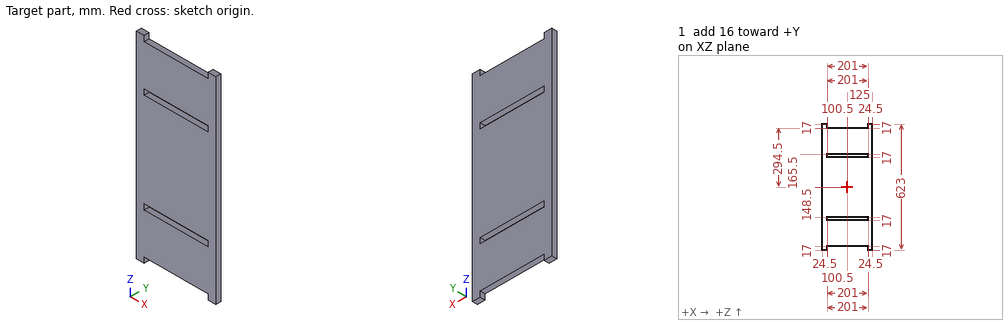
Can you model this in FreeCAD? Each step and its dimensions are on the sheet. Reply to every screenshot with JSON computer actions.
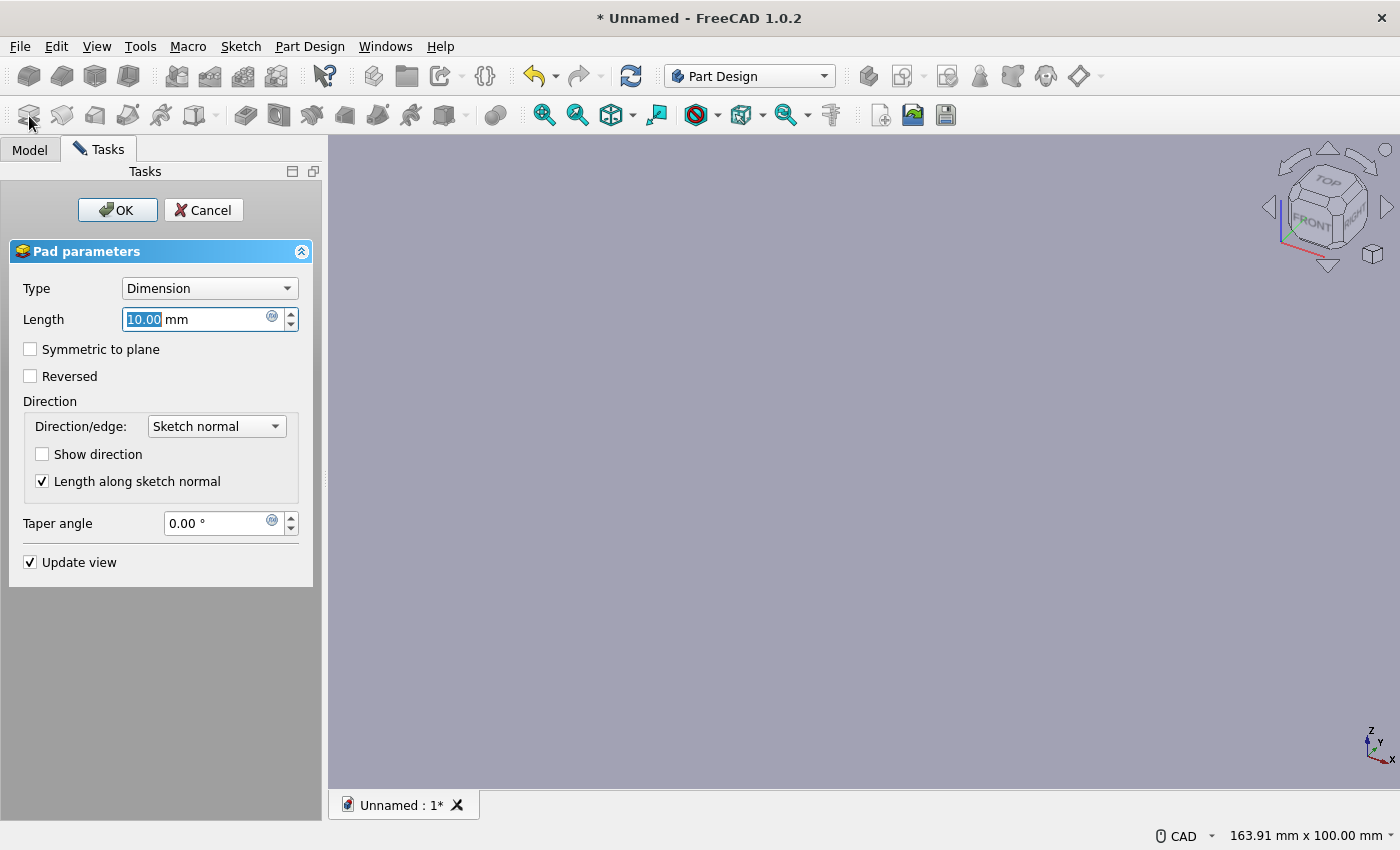
{"action": "type", "text": "16"}
{"action": "key", "text": "Tab"}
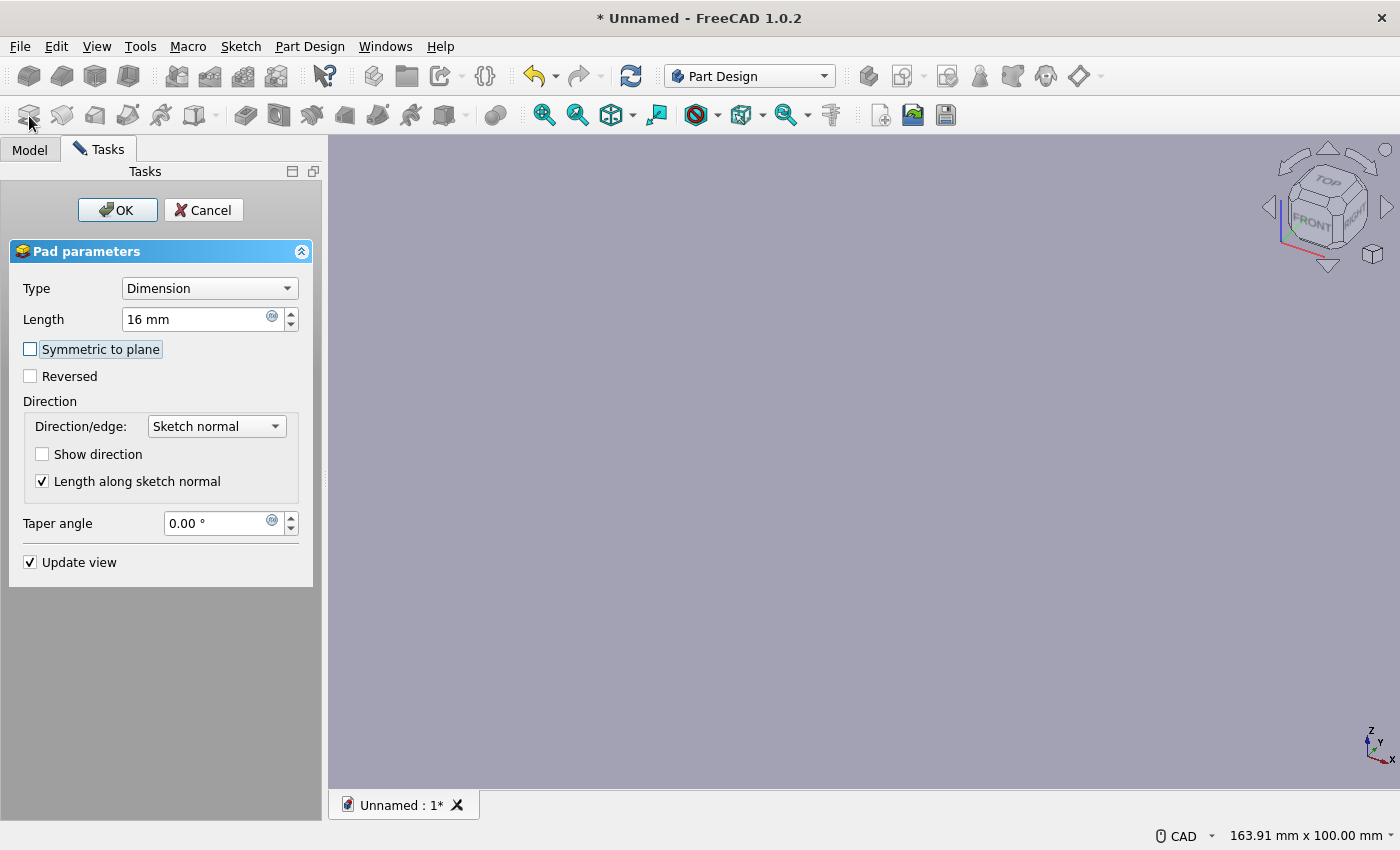
{"action": "left_click", "coordinate": [31, 376]}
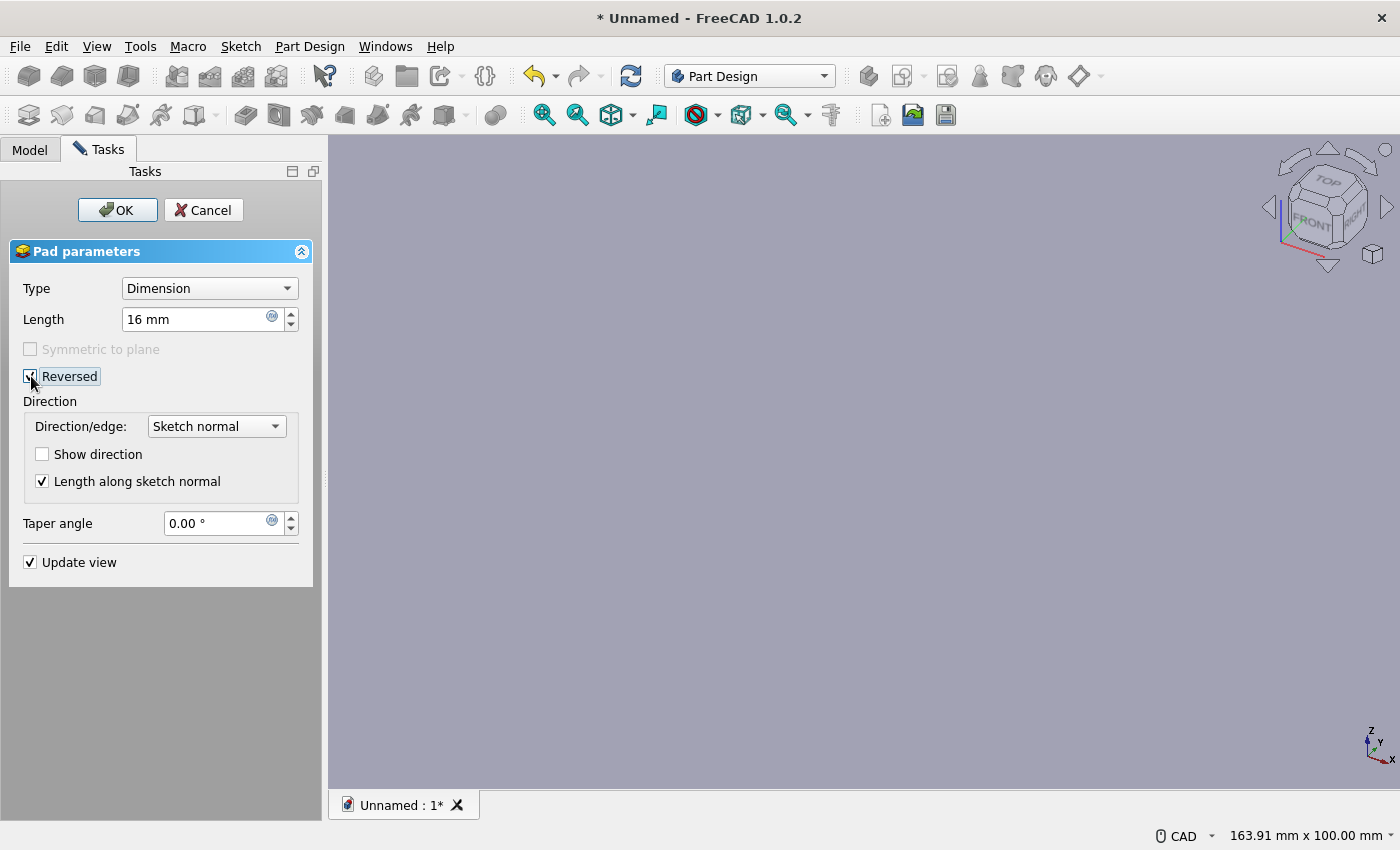
{"action": "left_click", "coordinate": [118, 210]}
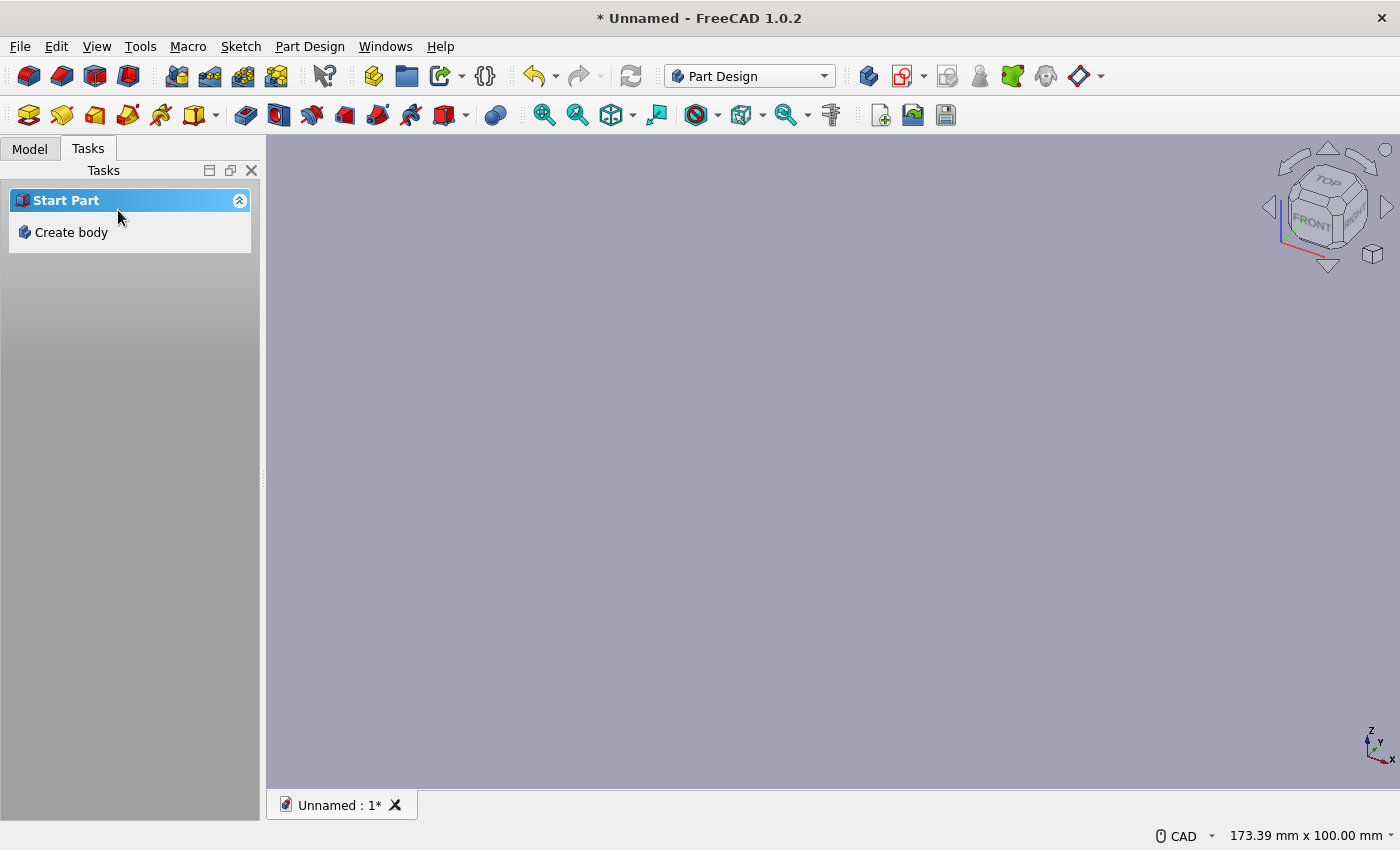
{"action": "key", "text": "0"}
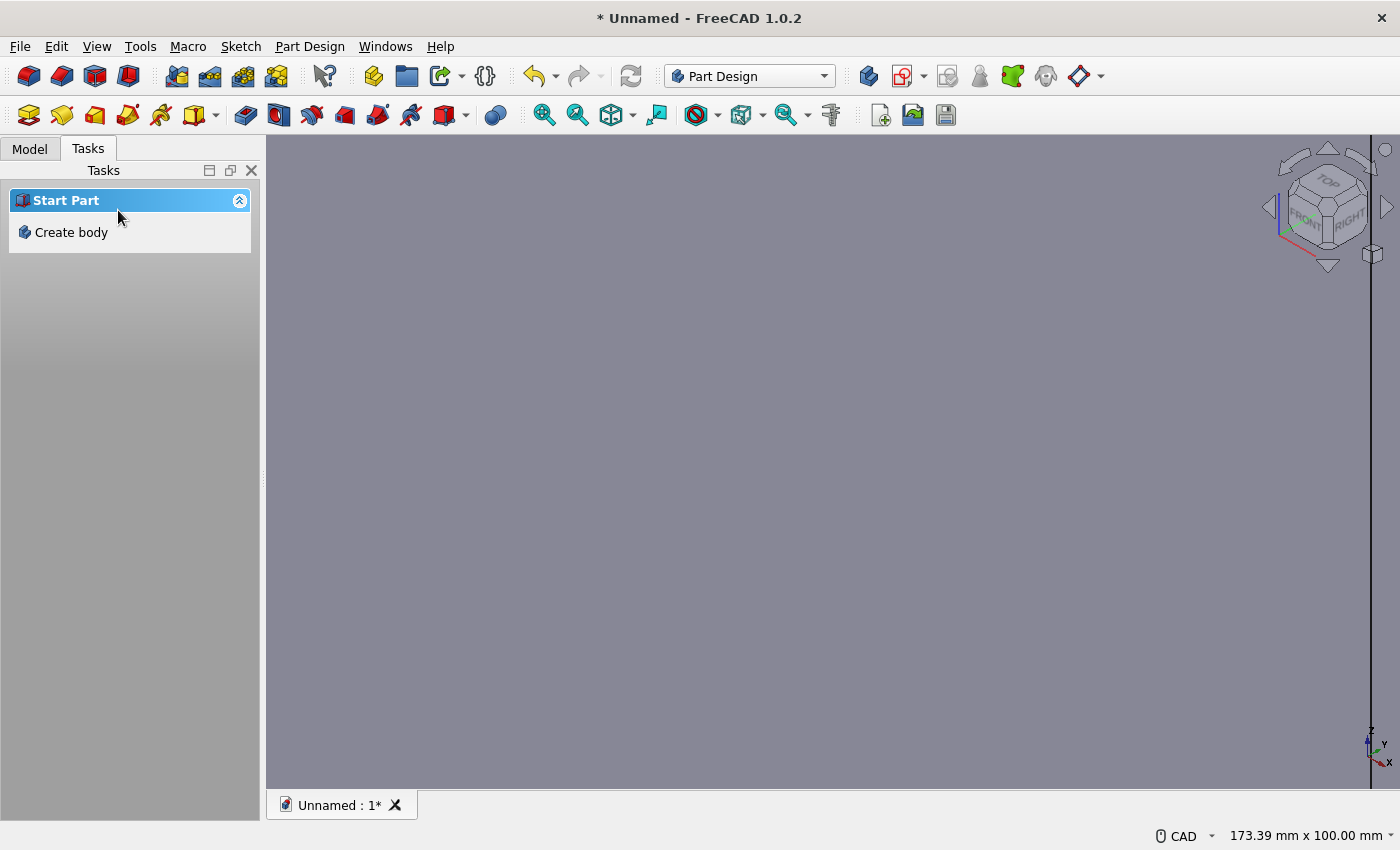
{"action": "left_click", "coordinate": [545, 116]}